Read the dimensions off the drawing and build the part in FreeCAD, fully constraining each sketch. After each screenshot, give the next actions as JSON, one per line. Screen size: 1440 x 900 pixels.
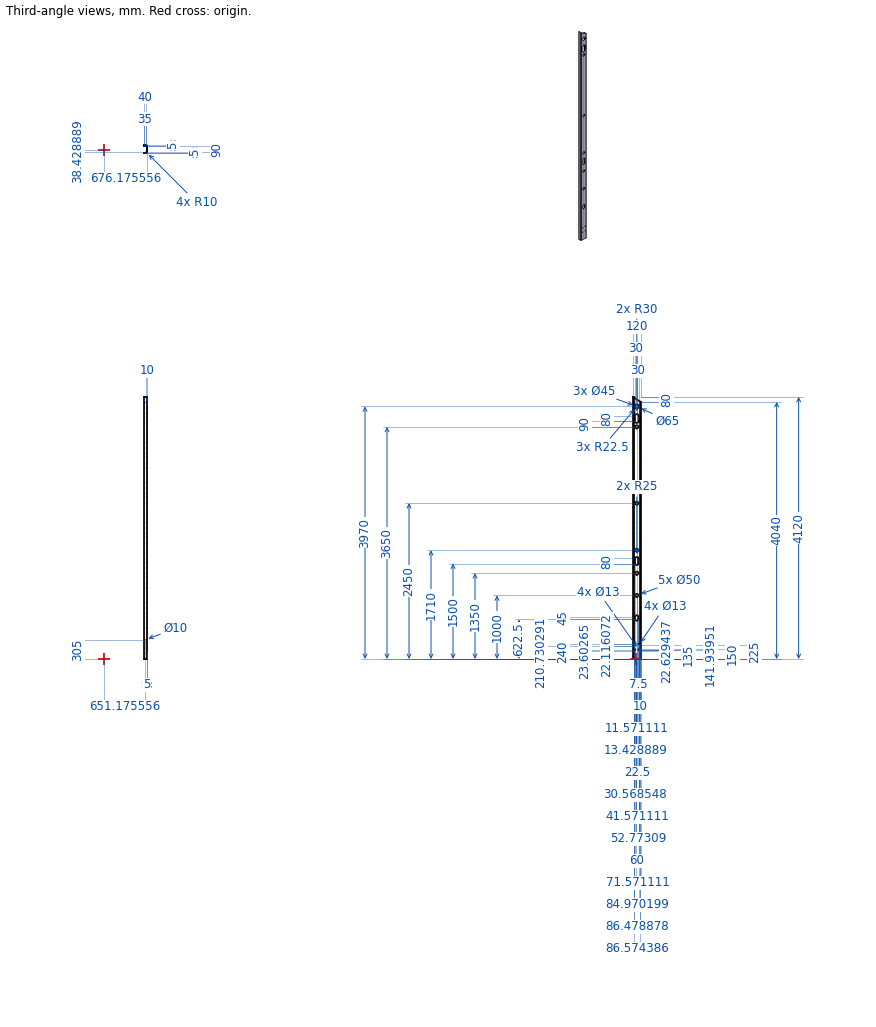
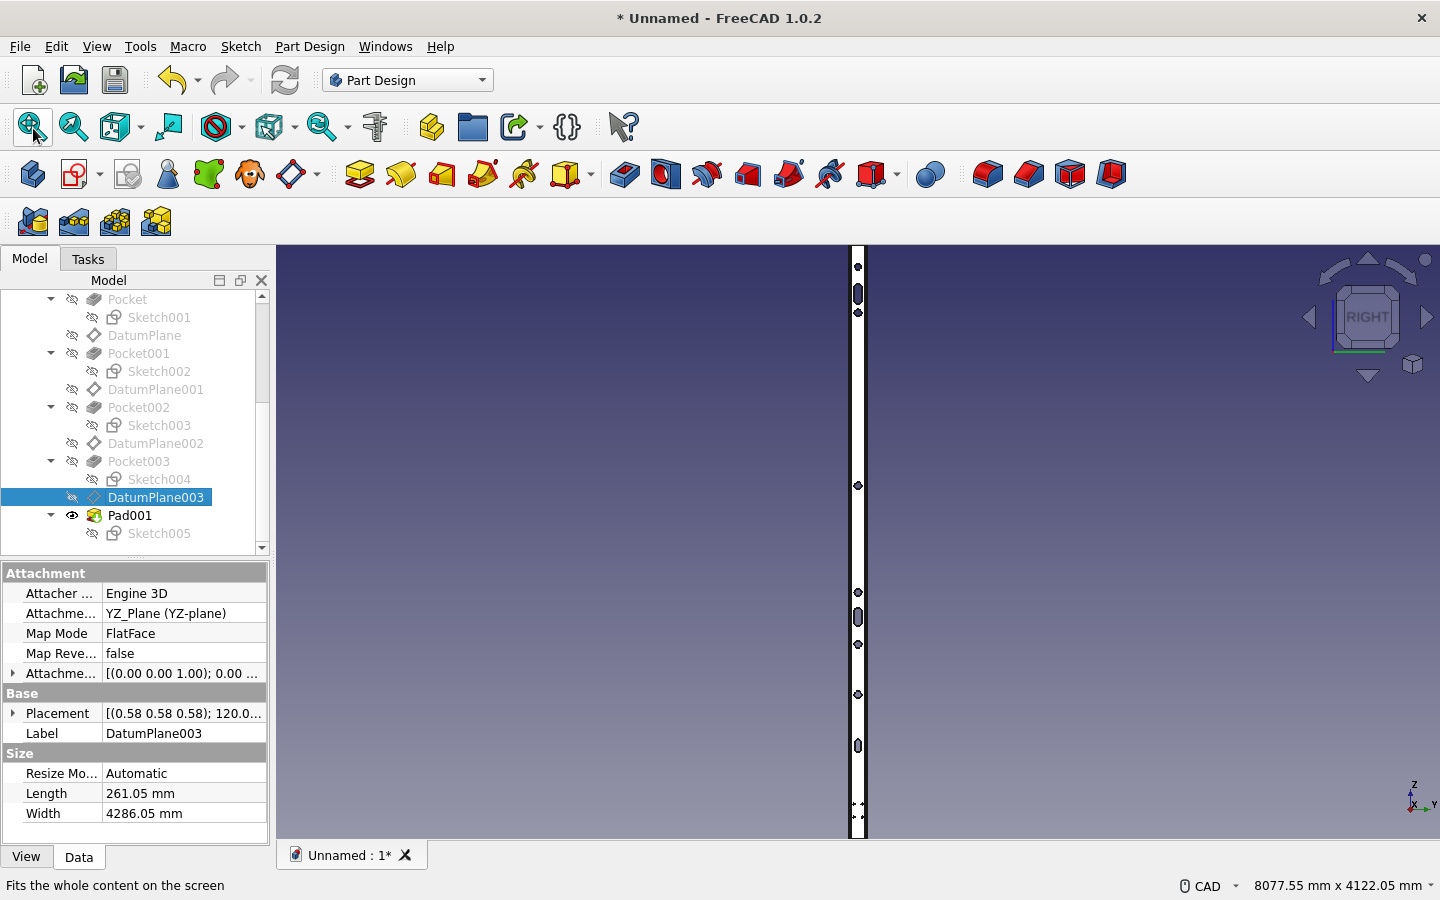
{"action": "key", "text": "v f"}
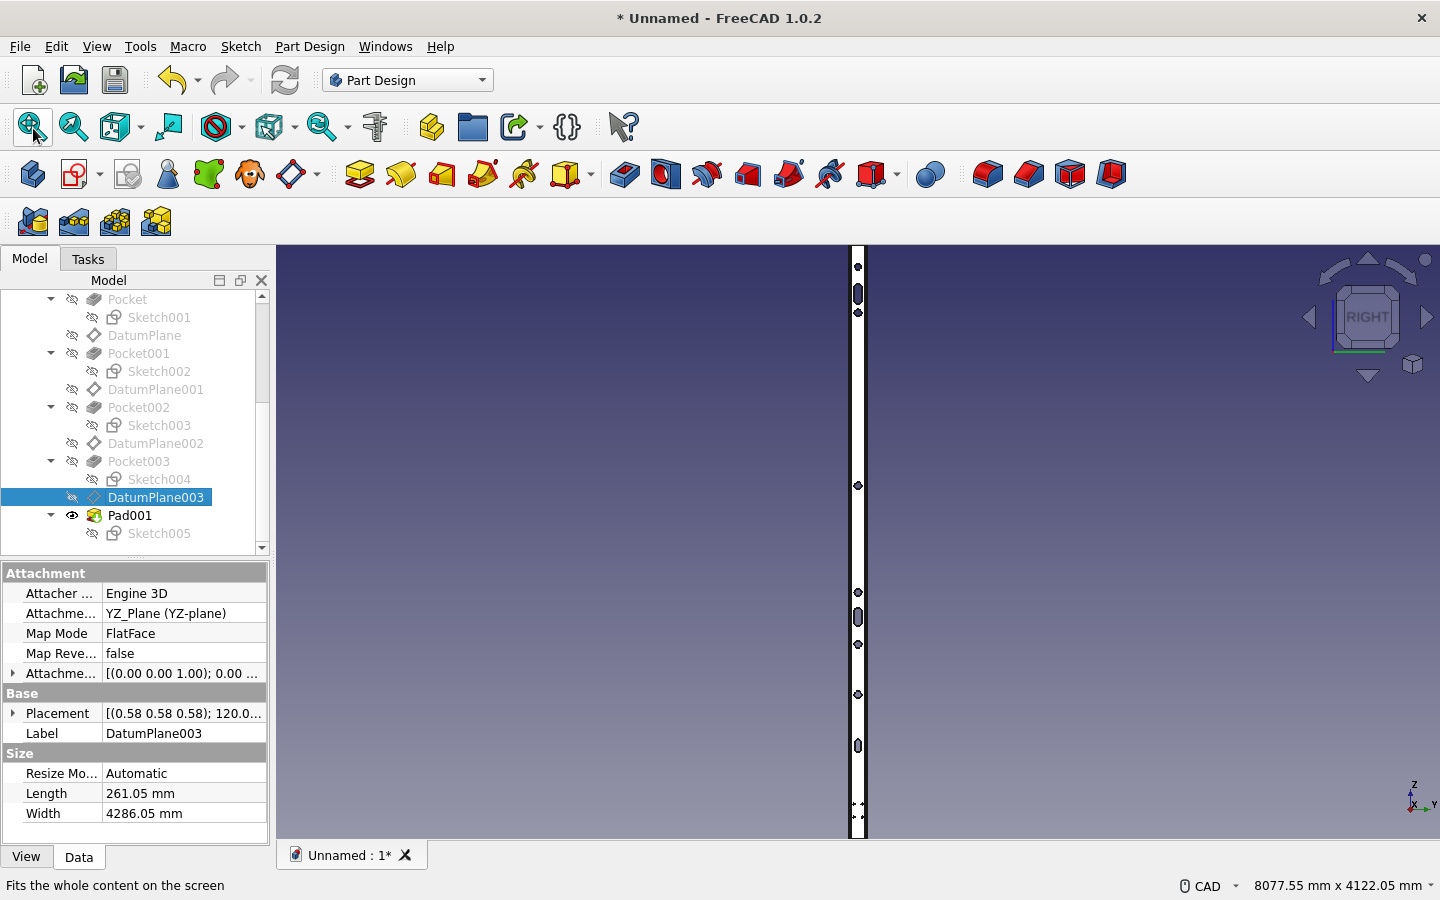
{"action": "key", "text": "2"}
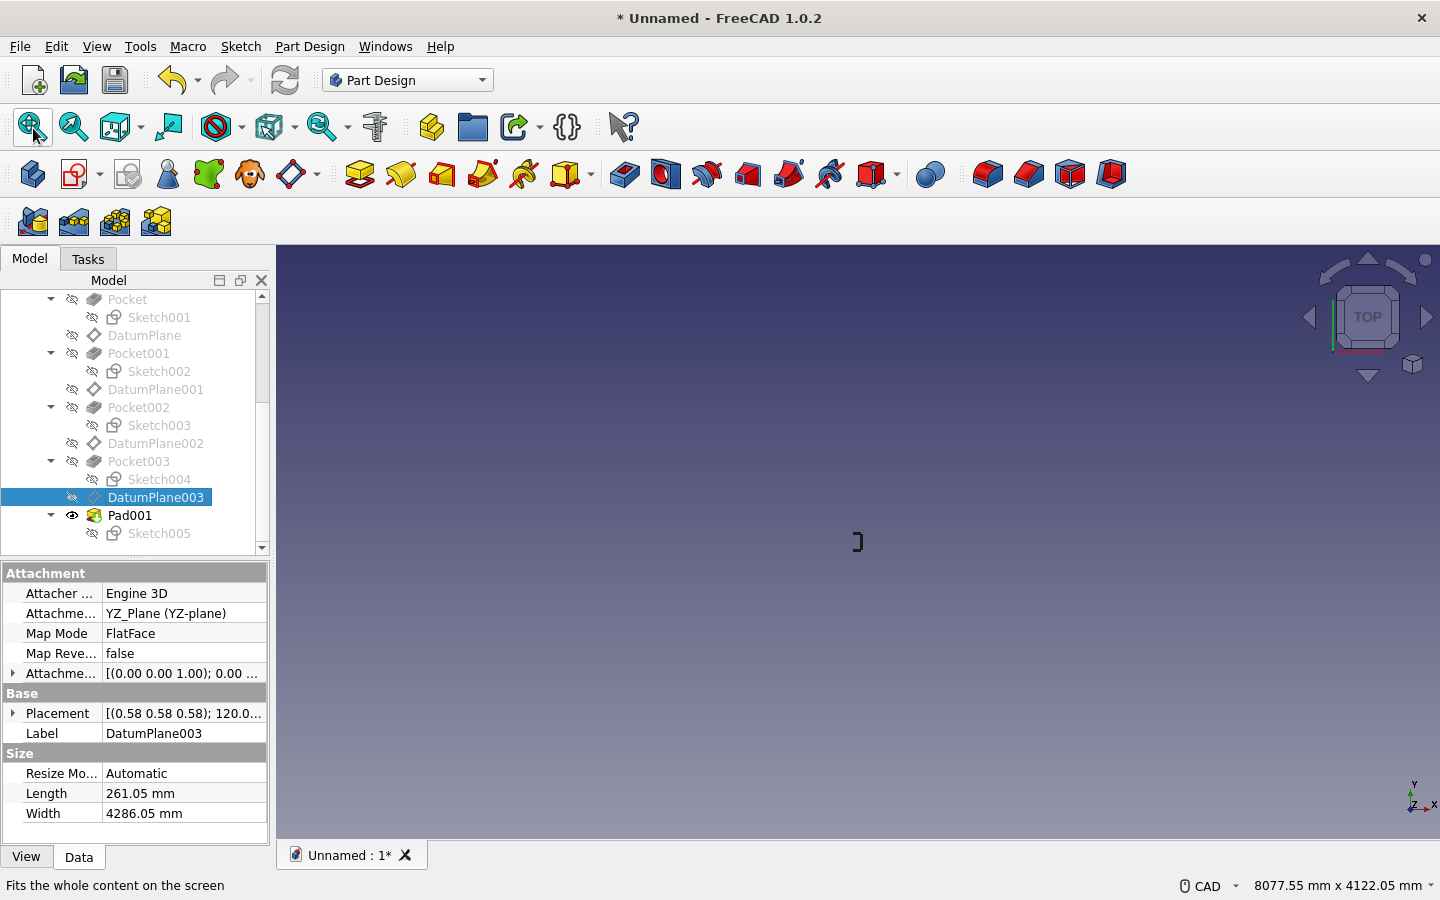
{"action": "key", "text": "v f"}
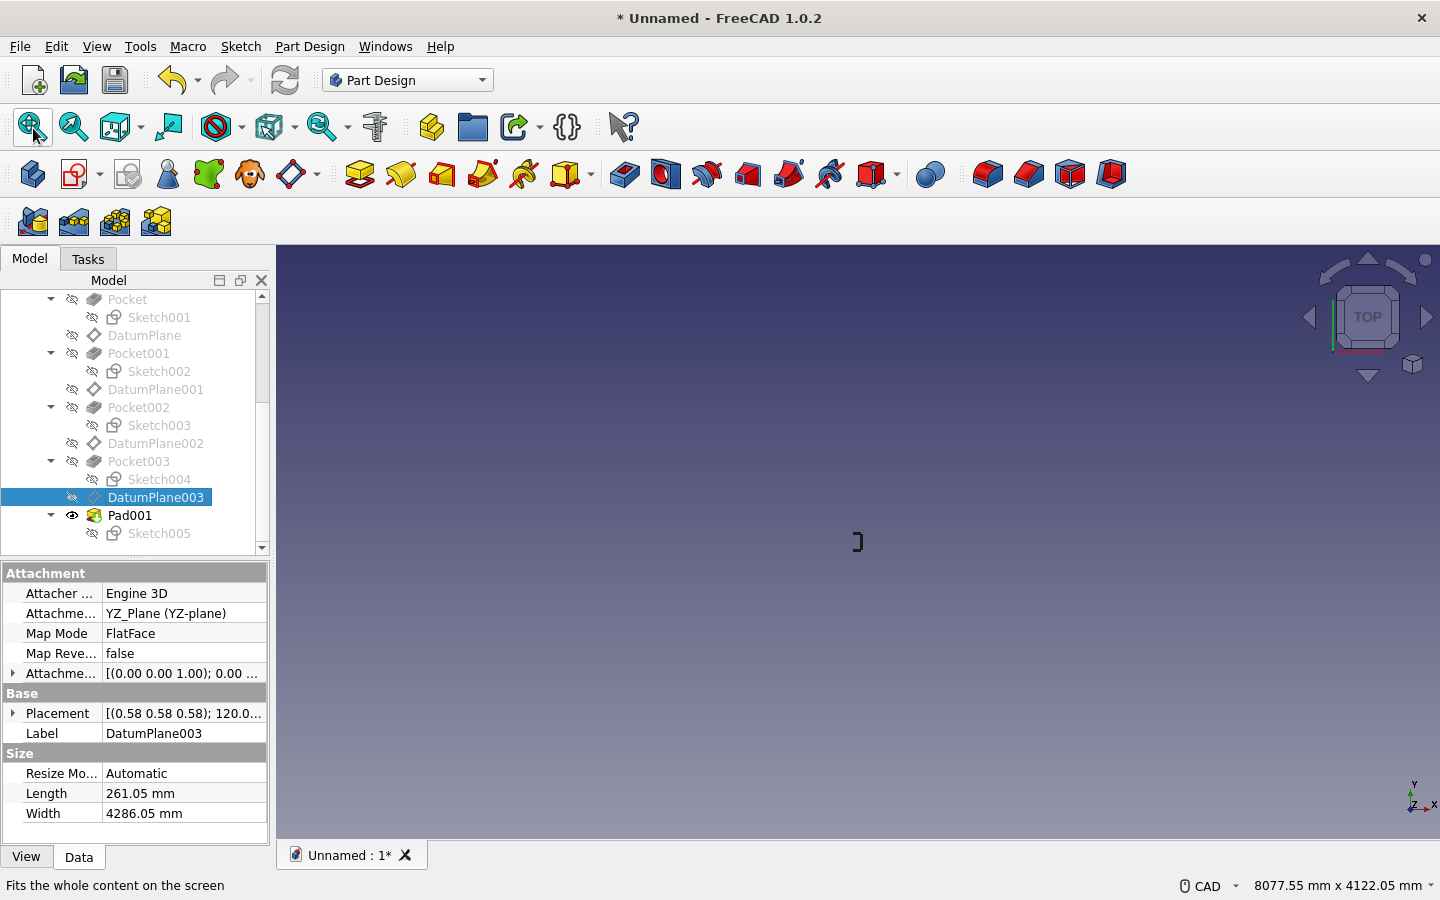
{"action": "scroll", "coordinate": [141, 421], "scroll_direction": "down", "scroll_amount": 3}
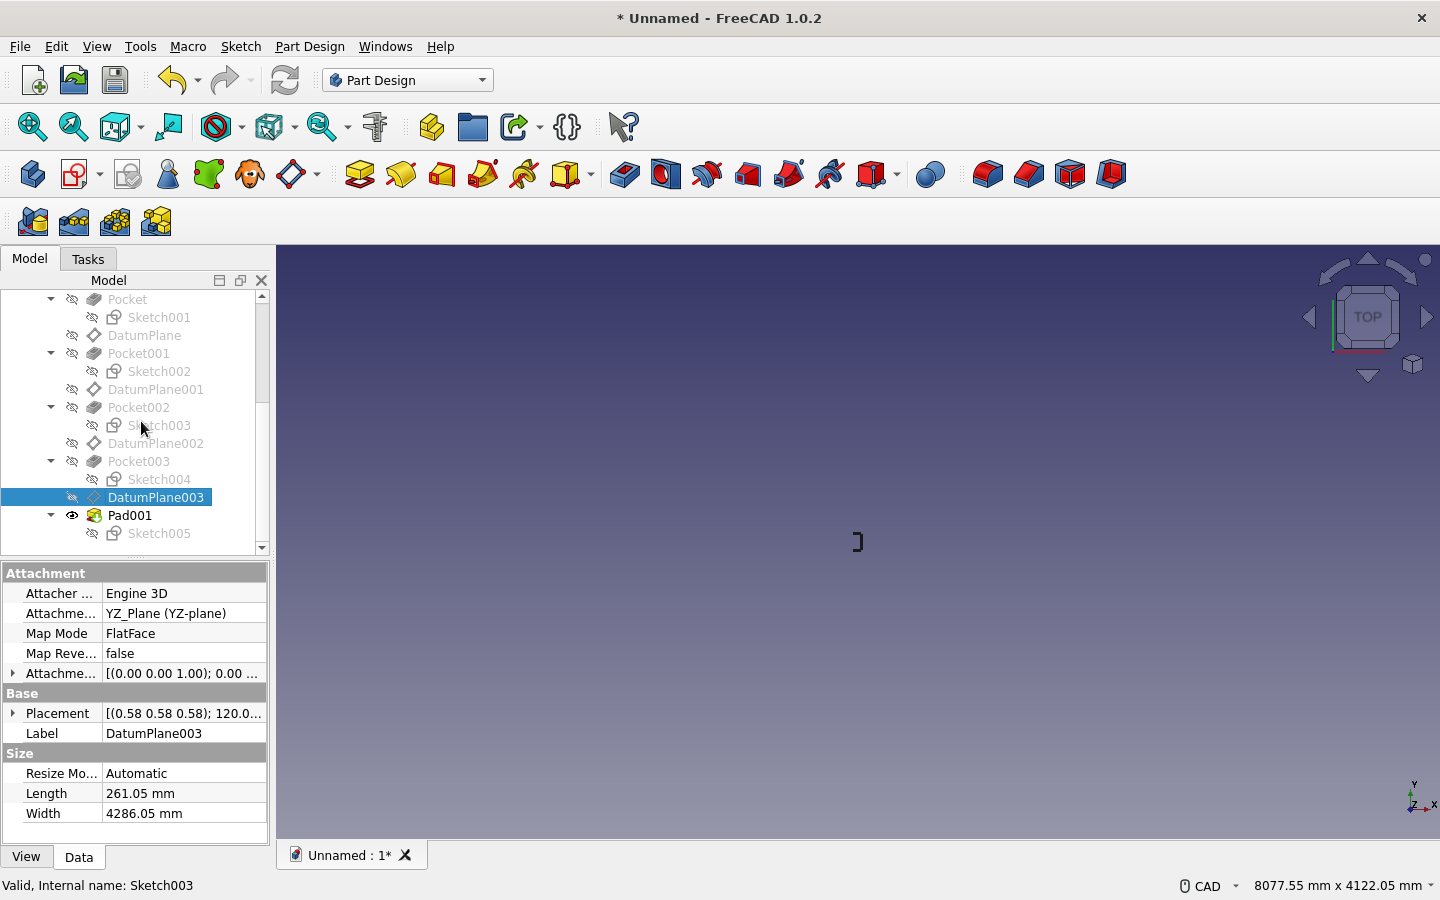
{"action": "scroll", "coordinate": [141, 421], "scroll_direction": "up", "scroll_amount": 15}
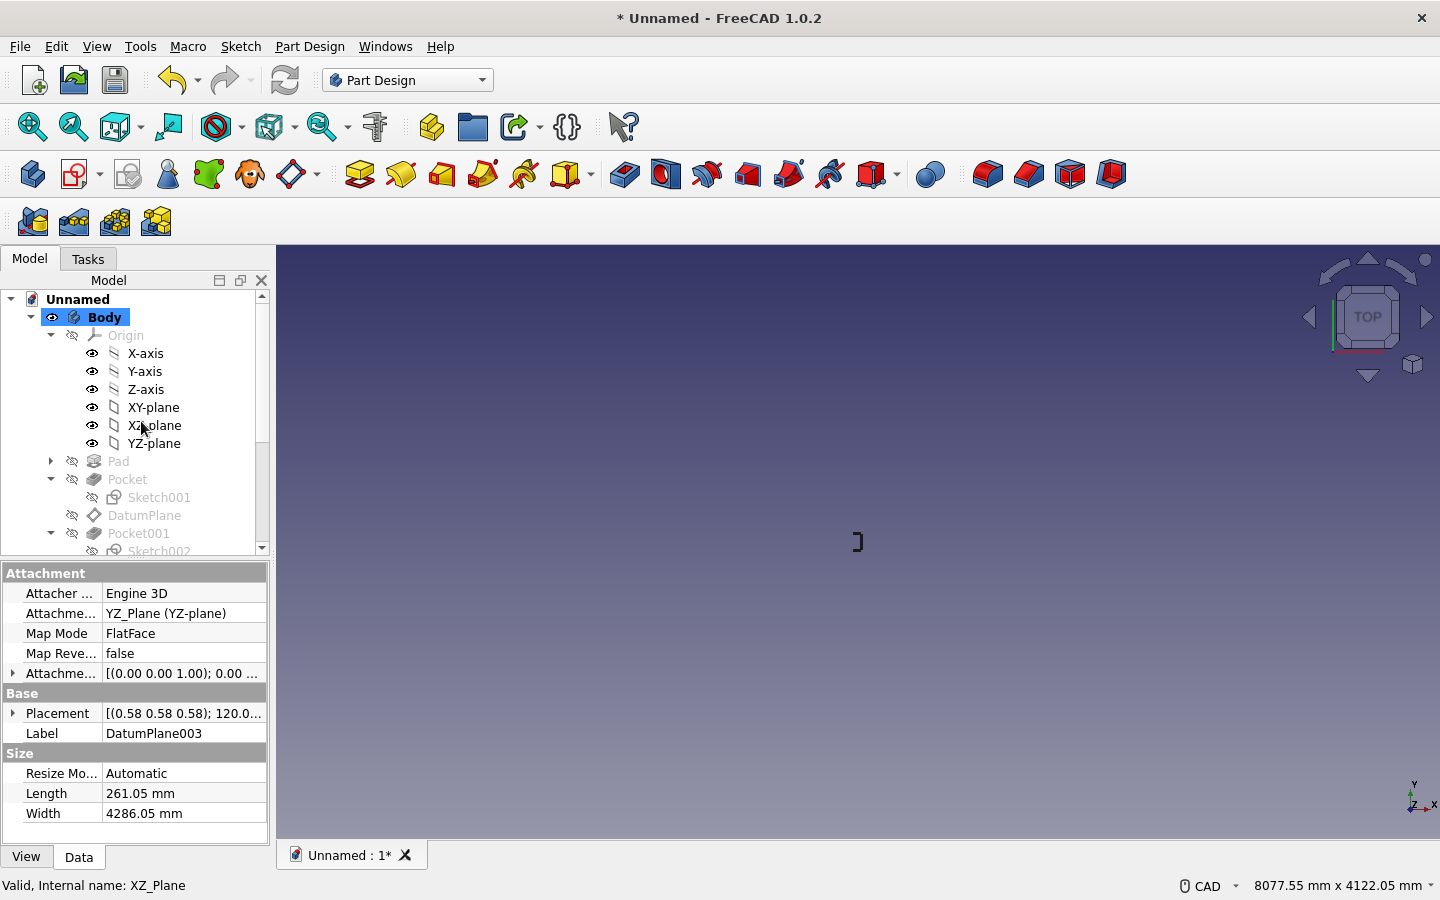
{"action": "left_click", "coordinate": [137, 443]}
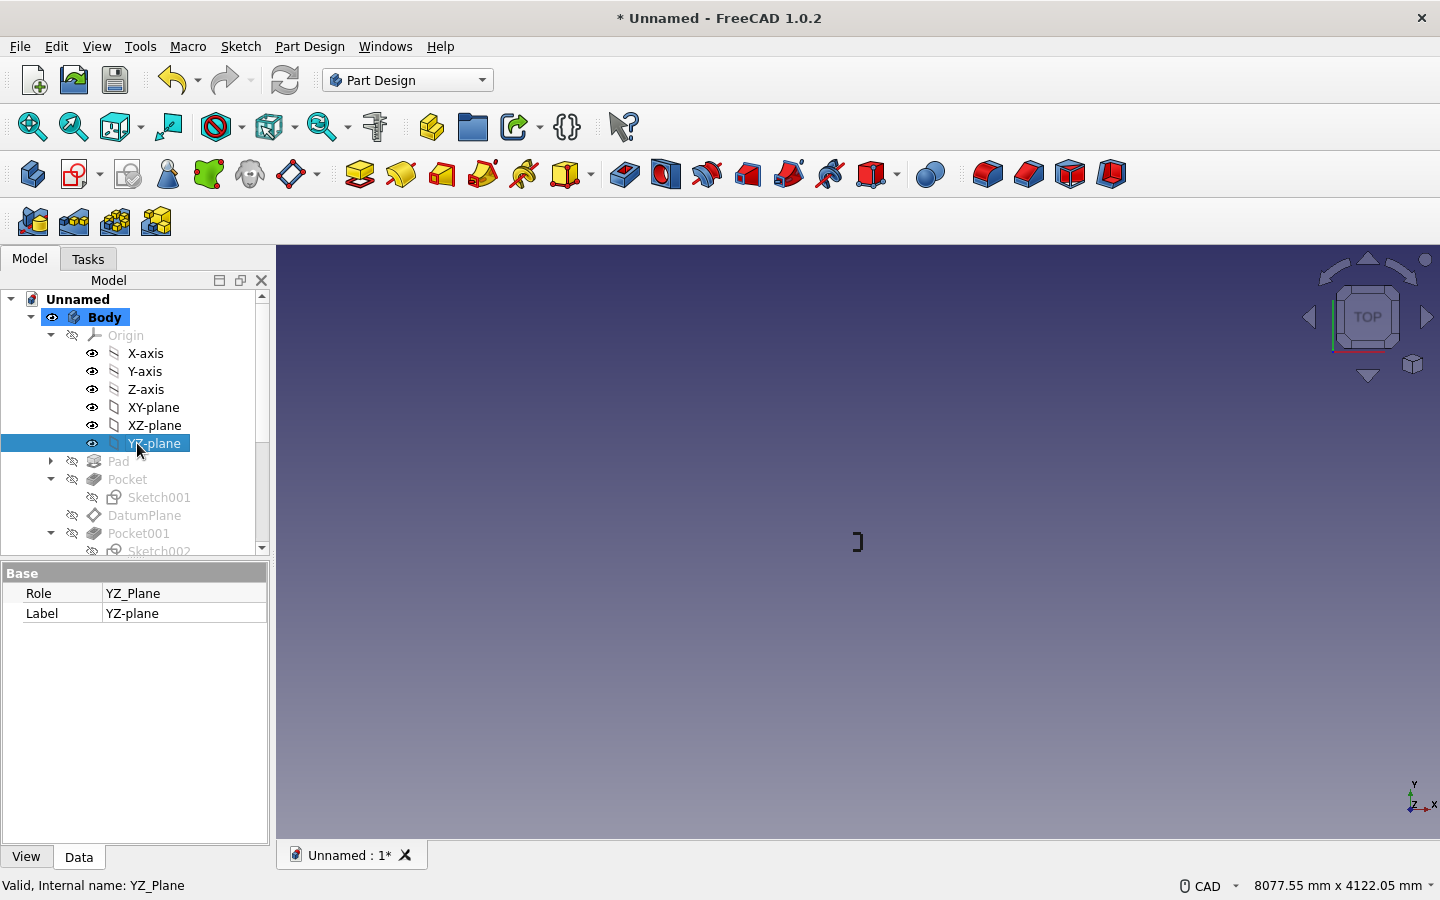
{"action": "left_click", "coordinate": [290, 174]}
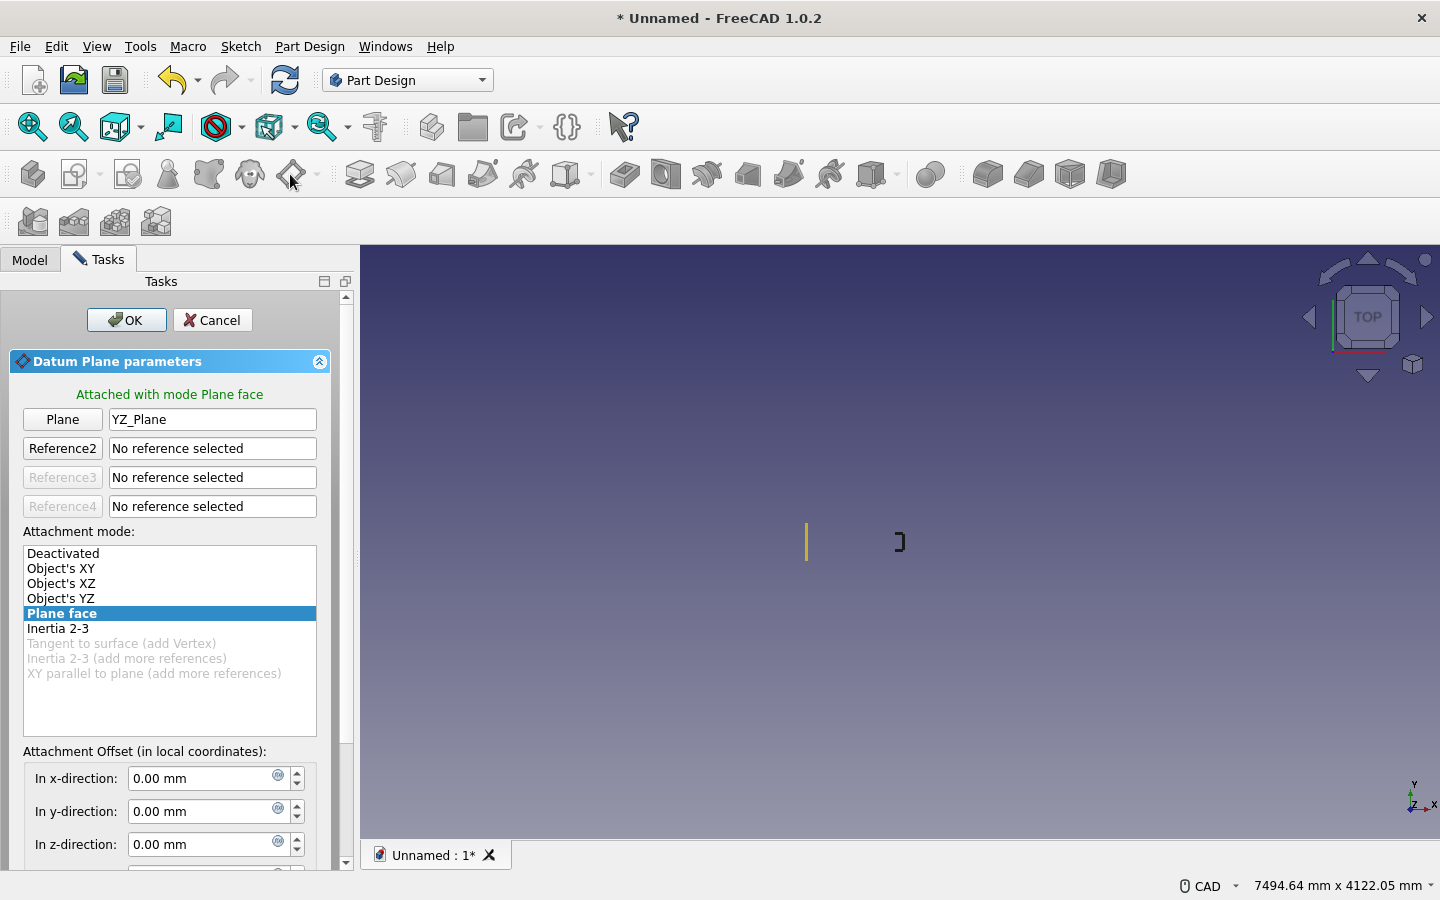
{"action": "triple_click", "coordinate": [210, 844]}